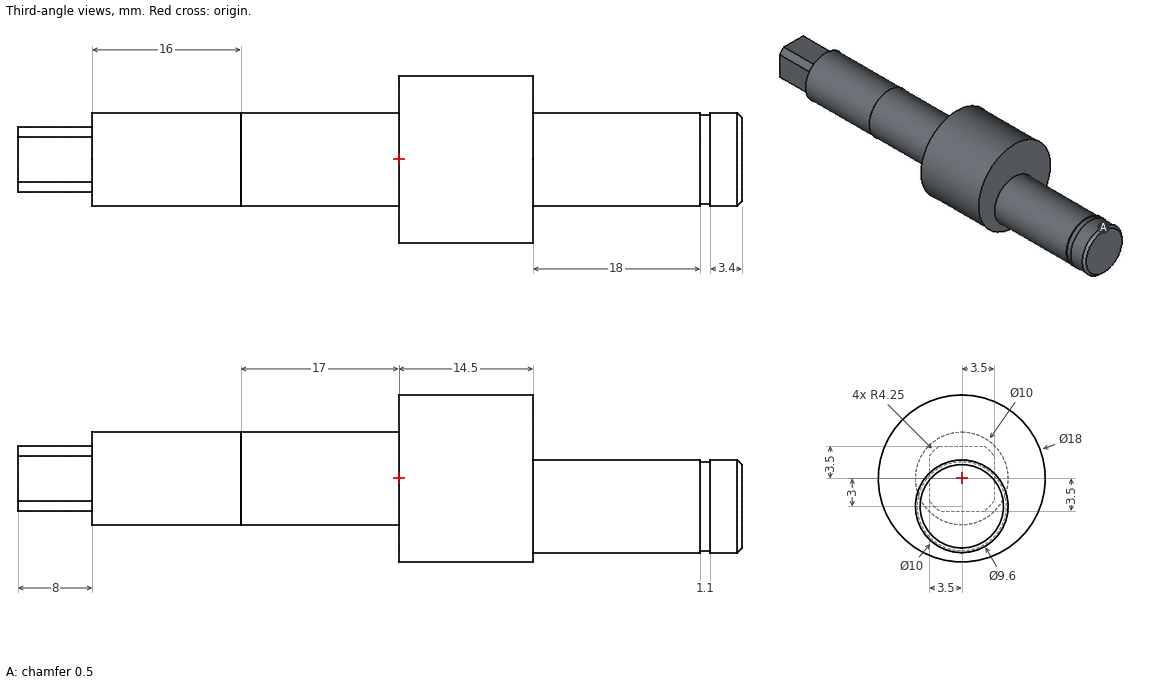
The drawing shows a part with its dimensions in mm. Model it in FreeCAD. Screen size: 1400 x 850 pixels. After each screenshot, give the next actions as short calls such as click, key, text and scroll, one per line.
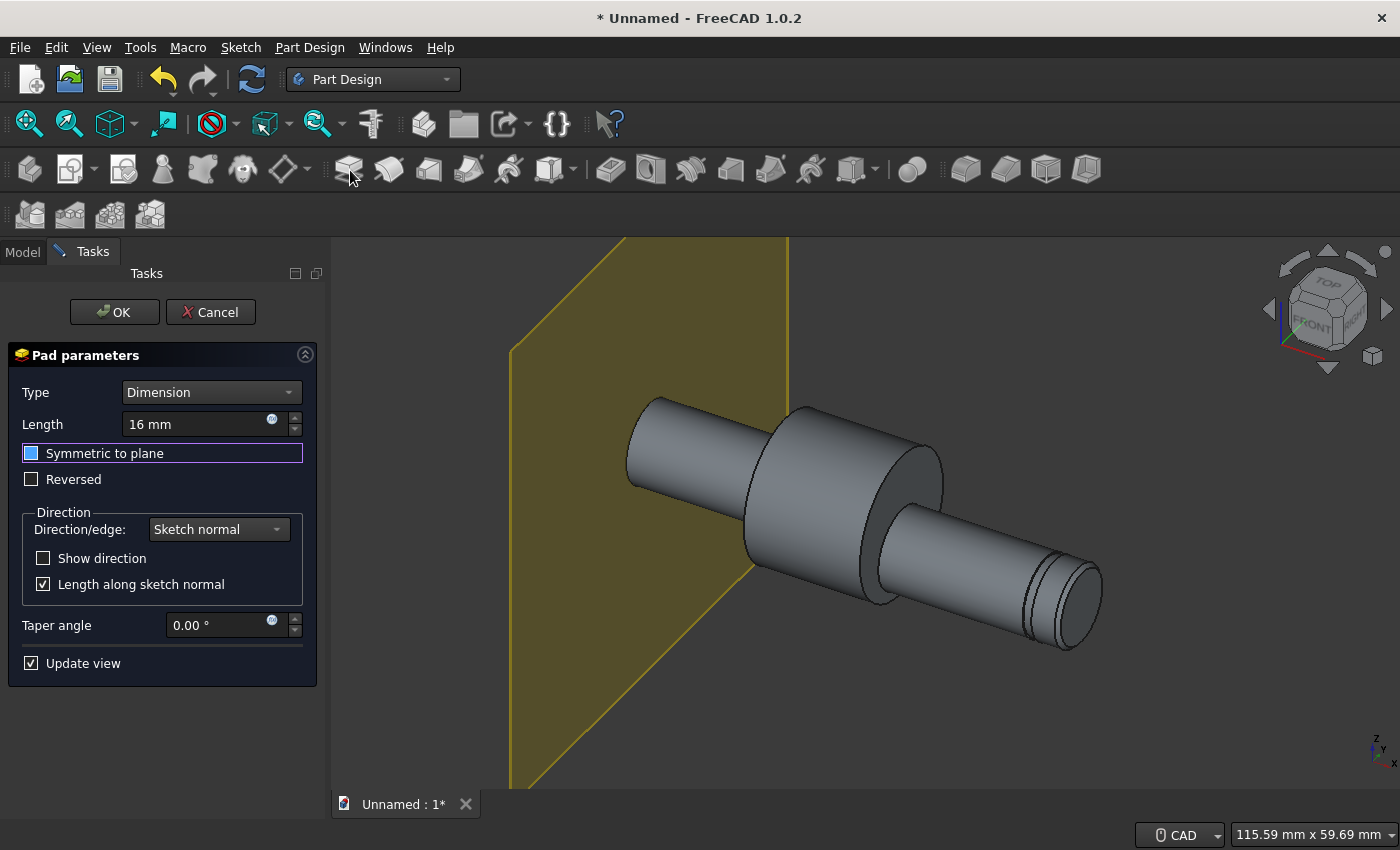
click(30, 479)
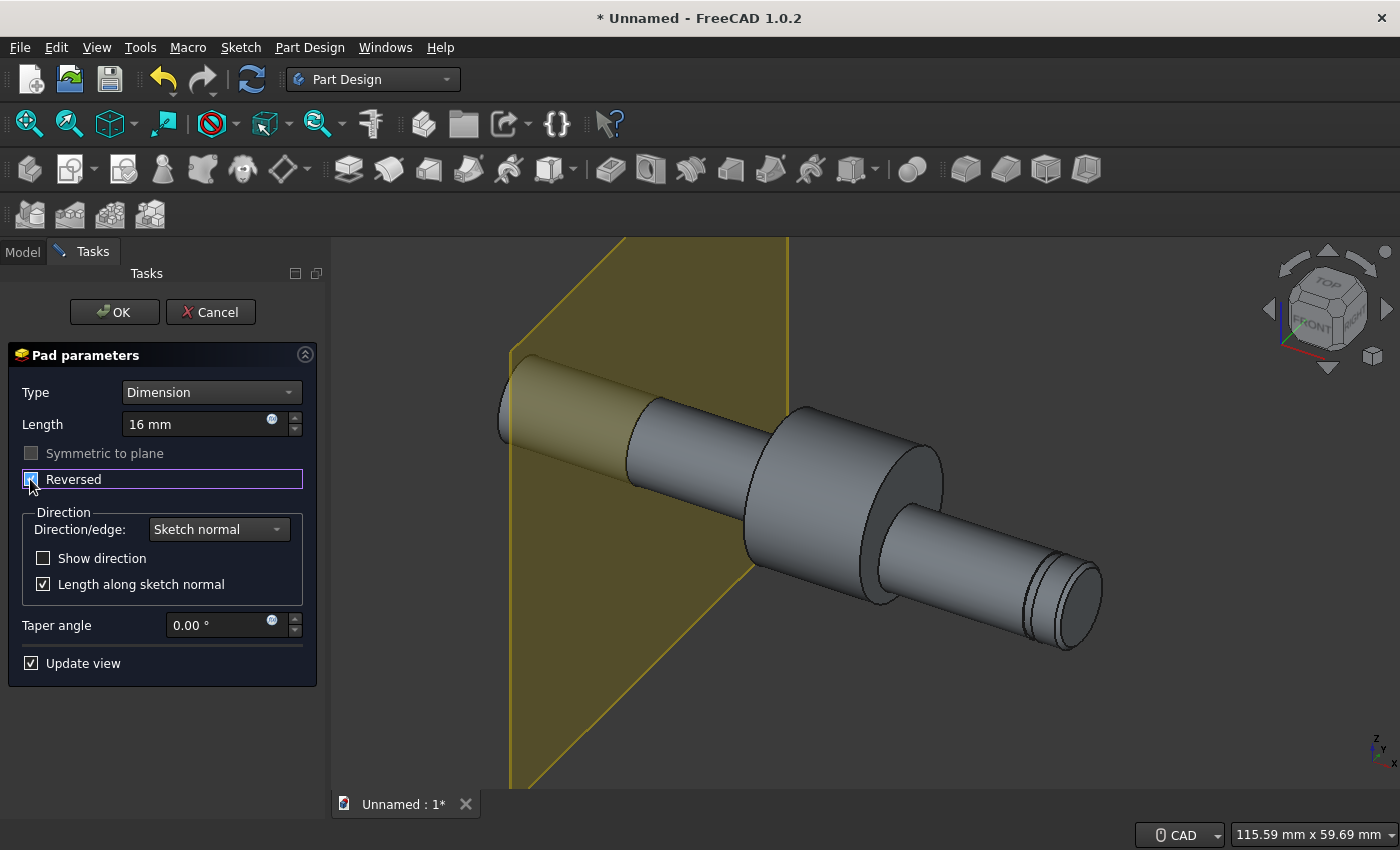
click(115, 312)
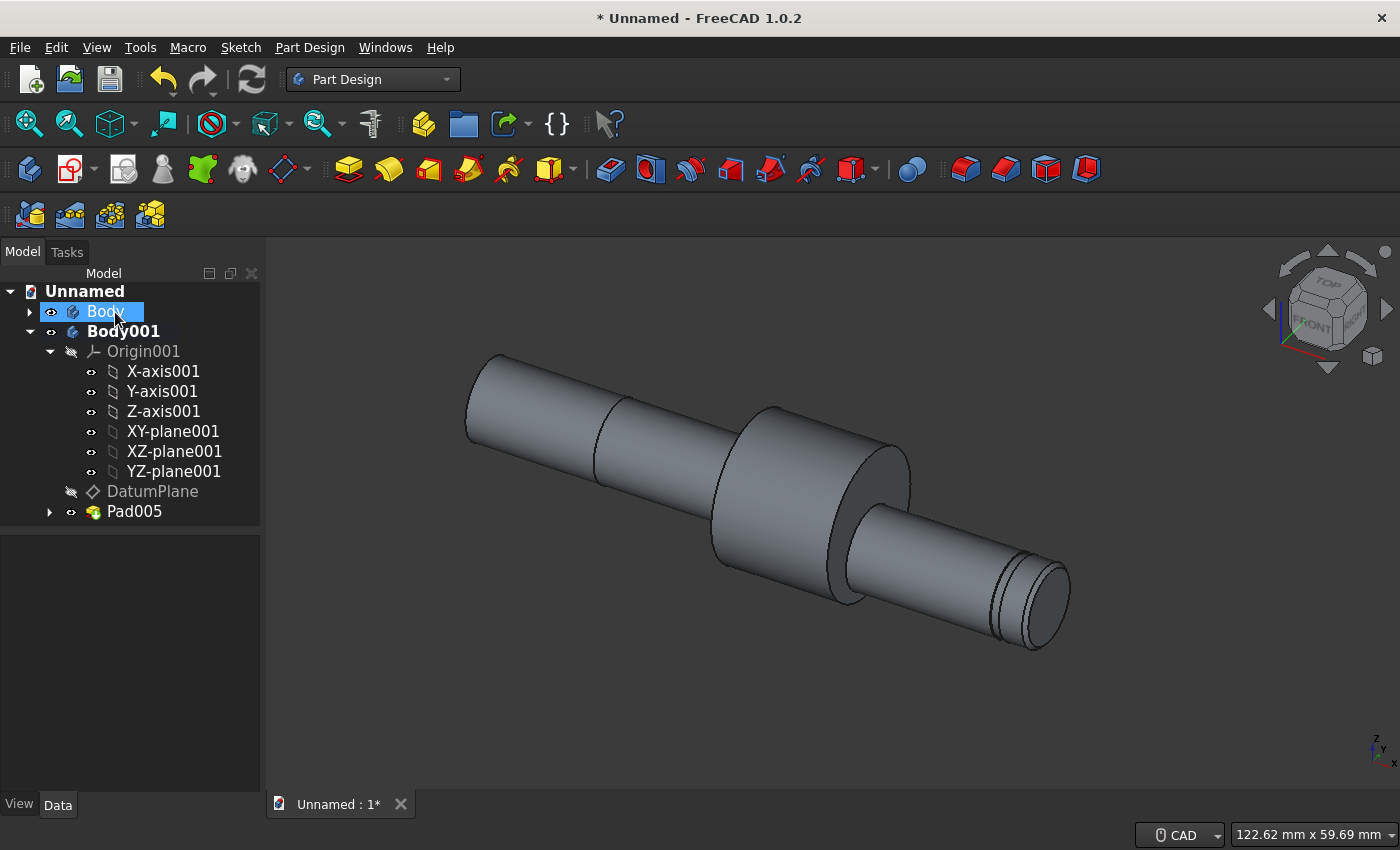
click(30, 124)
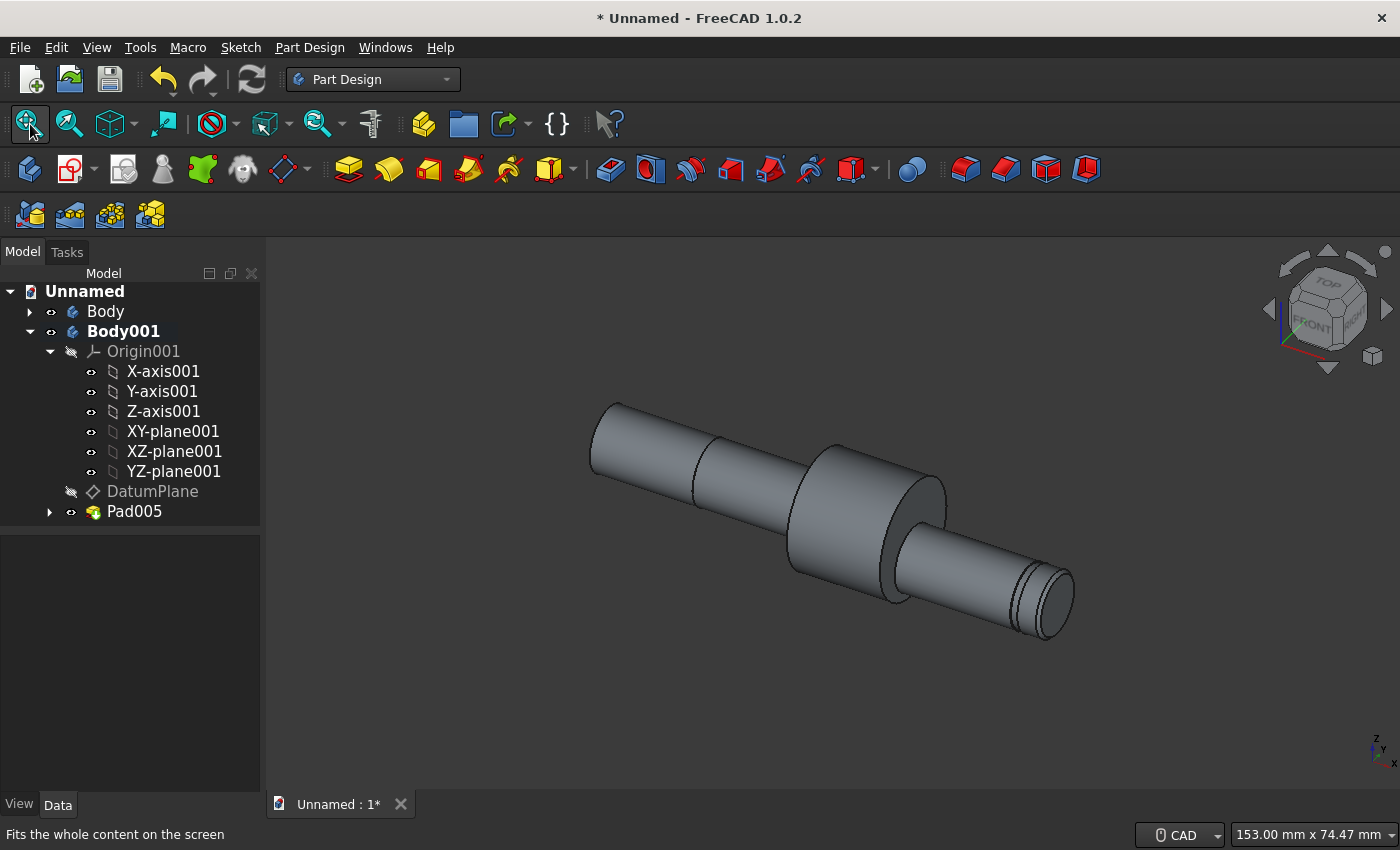
key(6)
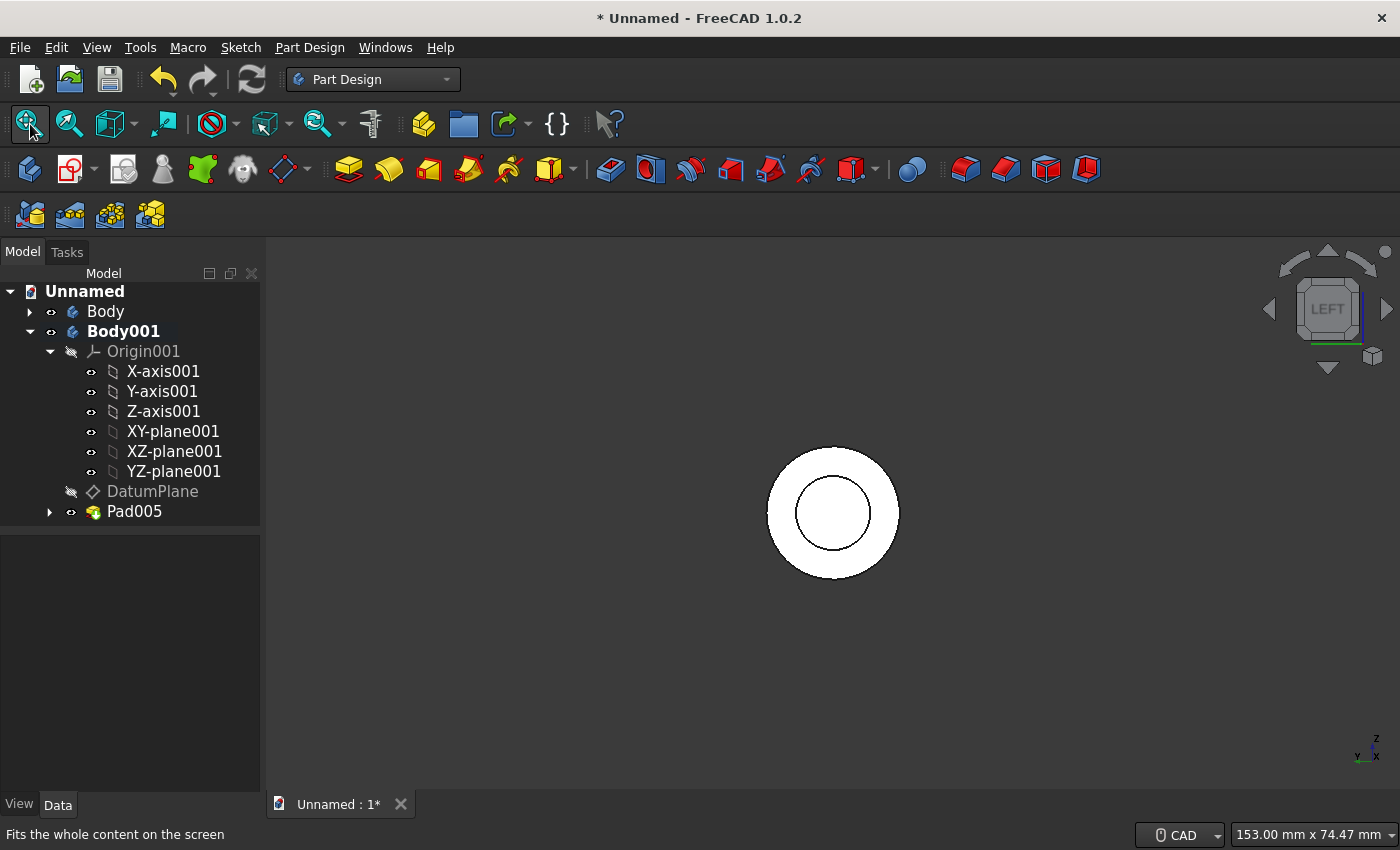
click(30, 124)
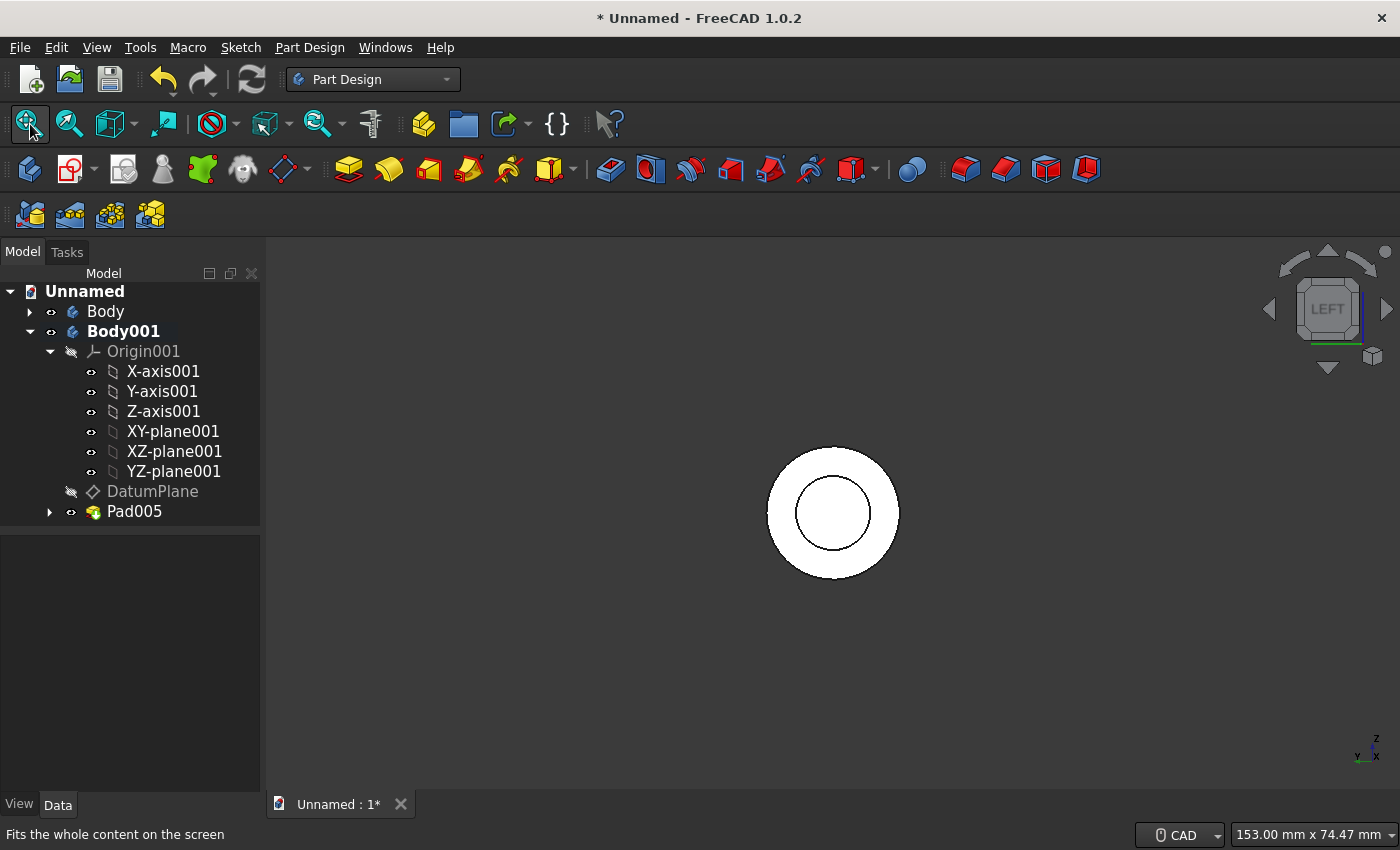
click(833, 512)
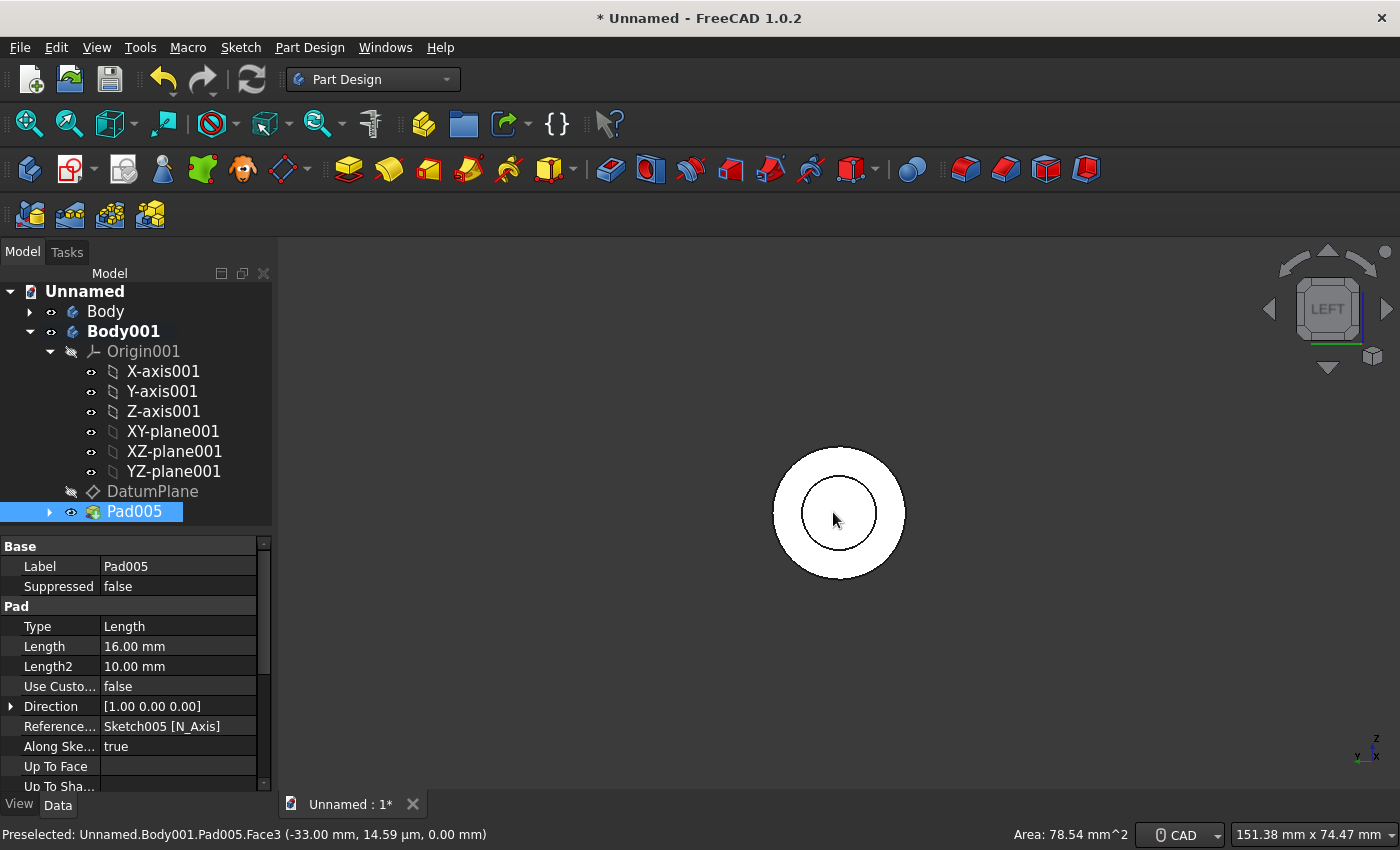
click(70, 170)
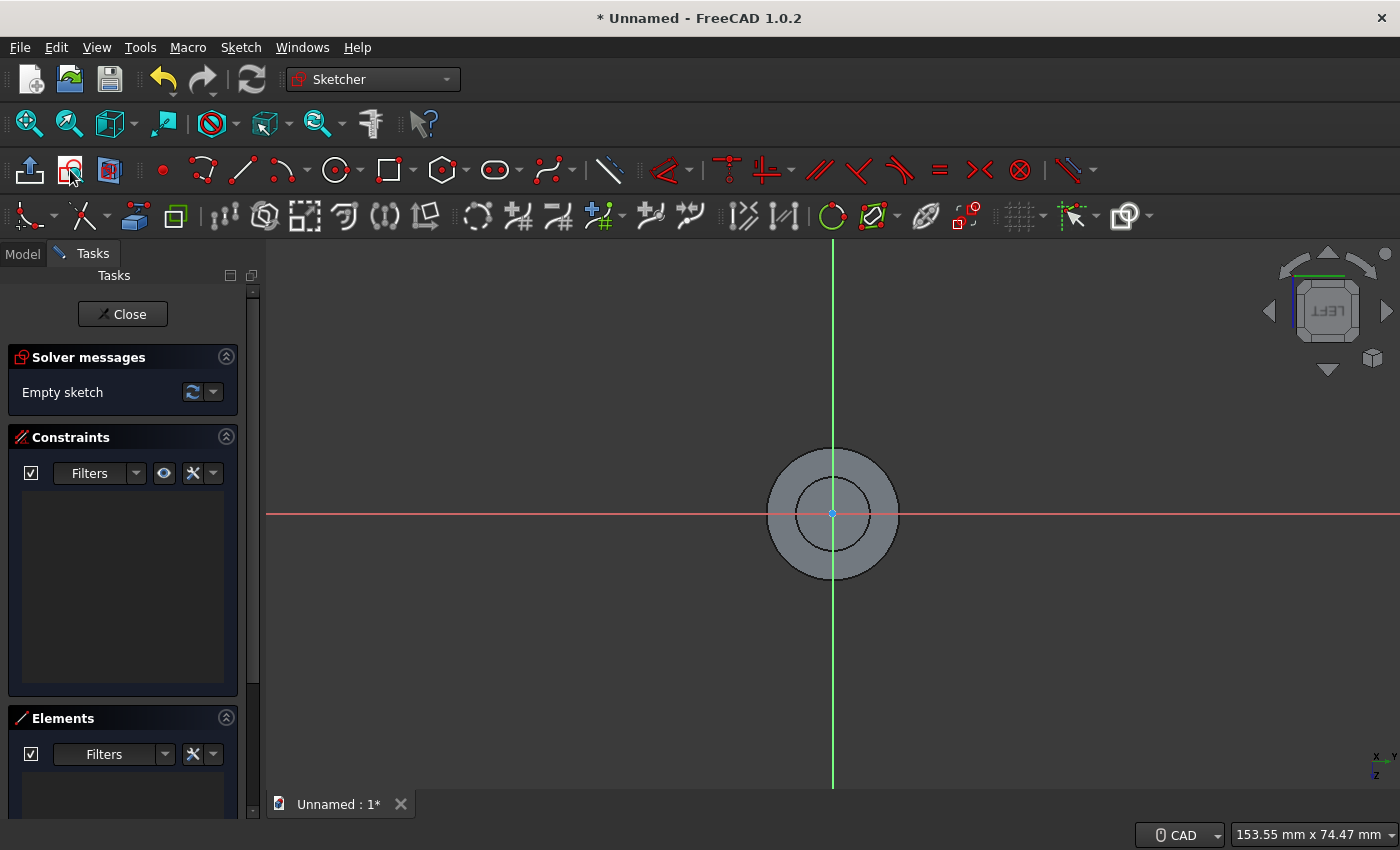
scroll(844, 514, up, 10)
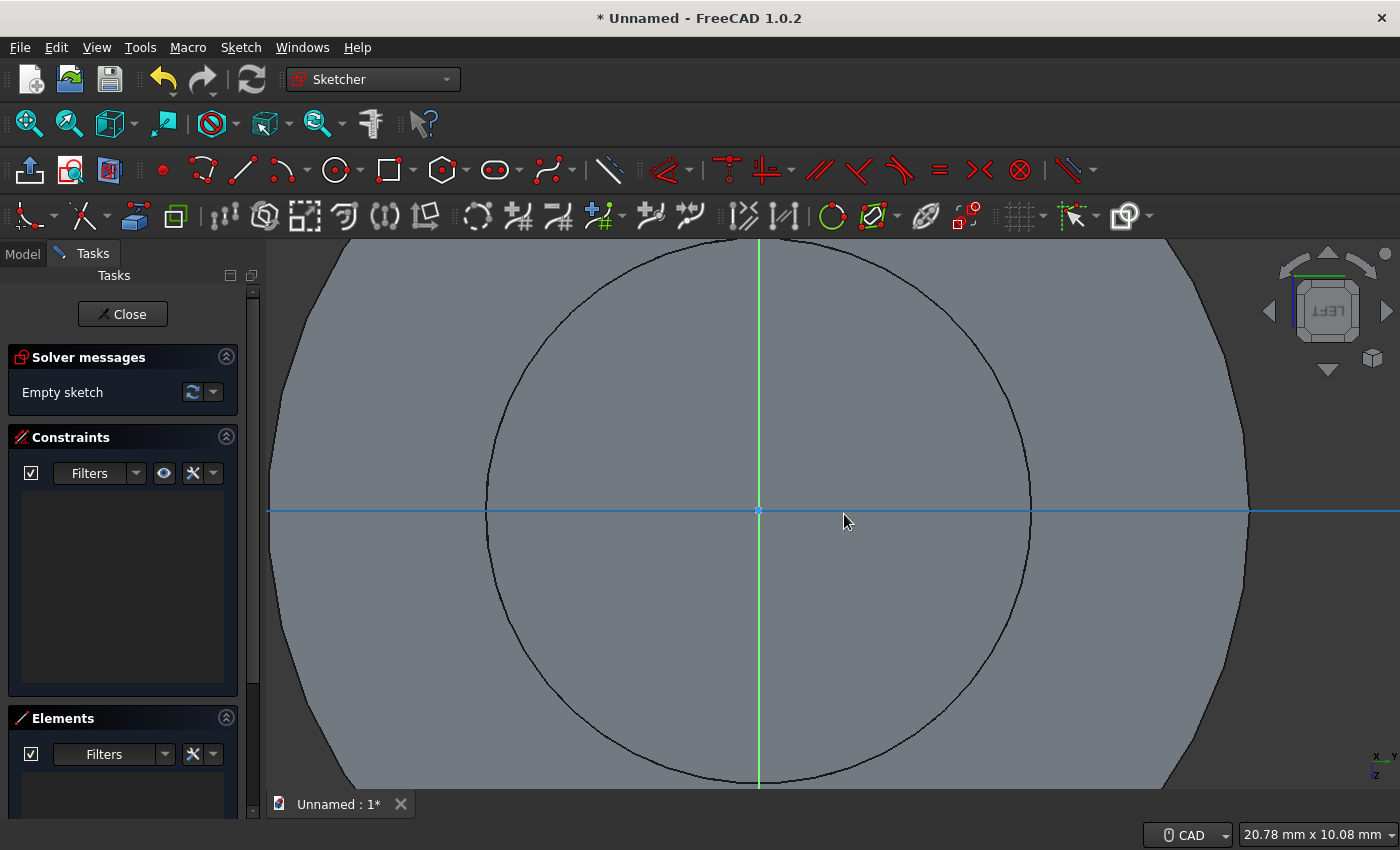
click(244, 170)